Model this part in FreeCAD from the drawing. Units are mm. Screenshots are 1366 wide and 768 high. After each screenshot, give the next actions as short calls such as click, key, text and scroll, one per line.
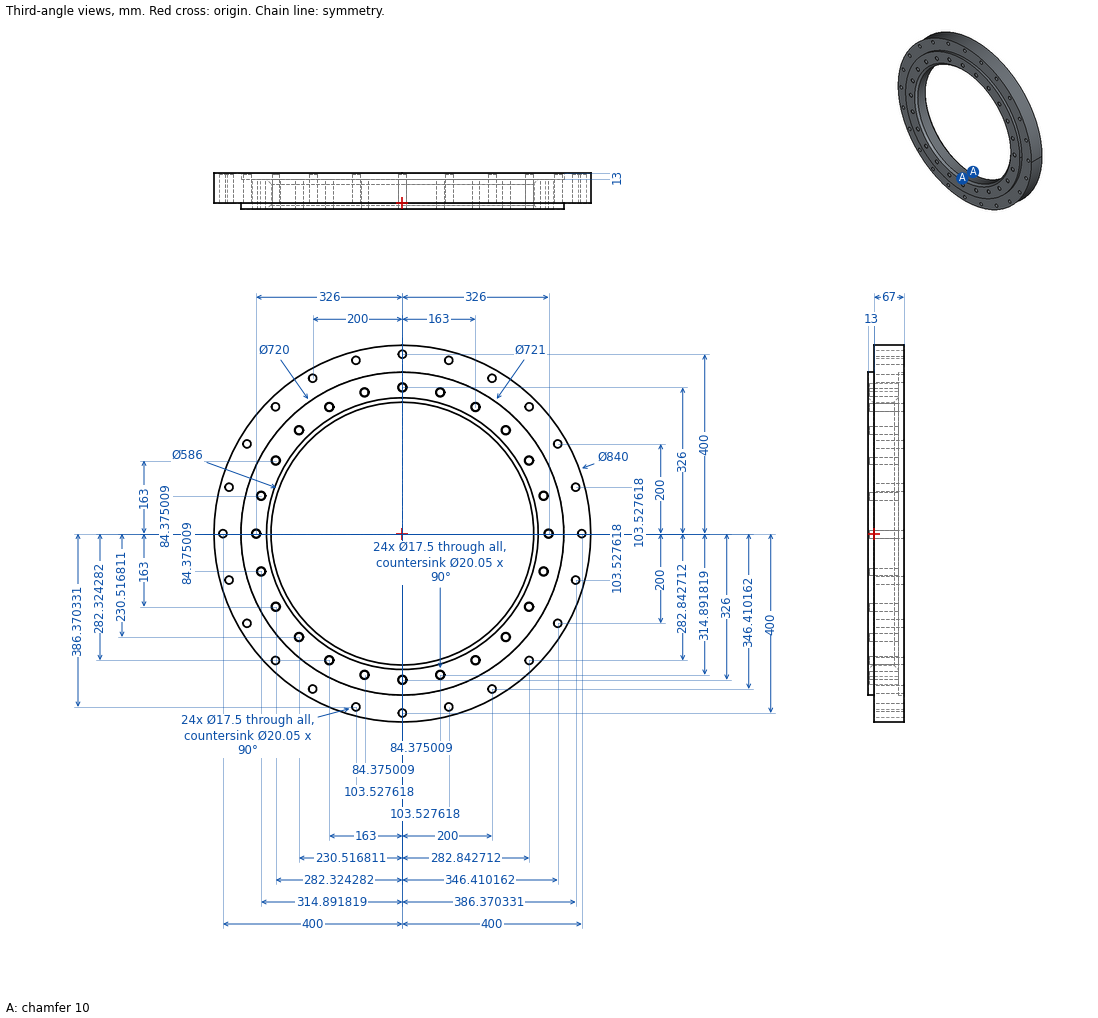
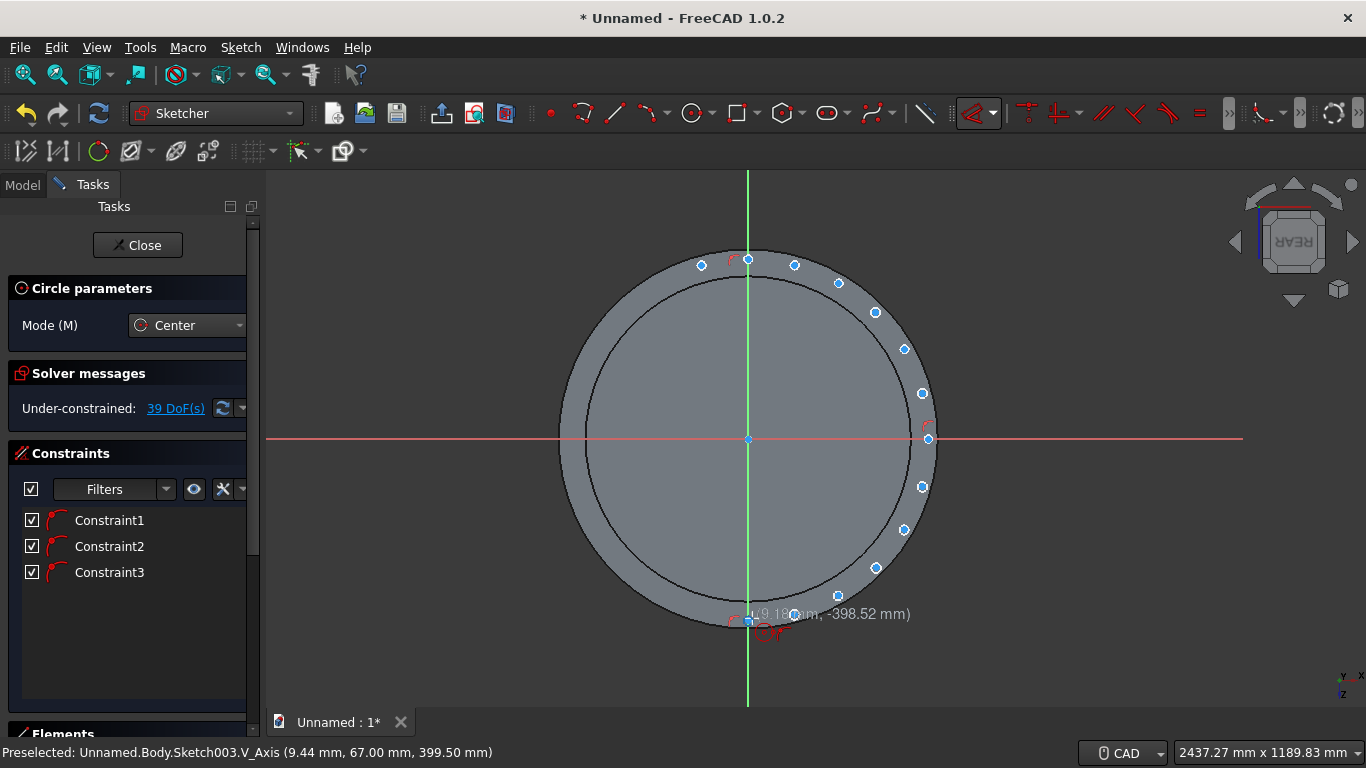
click(701, 613)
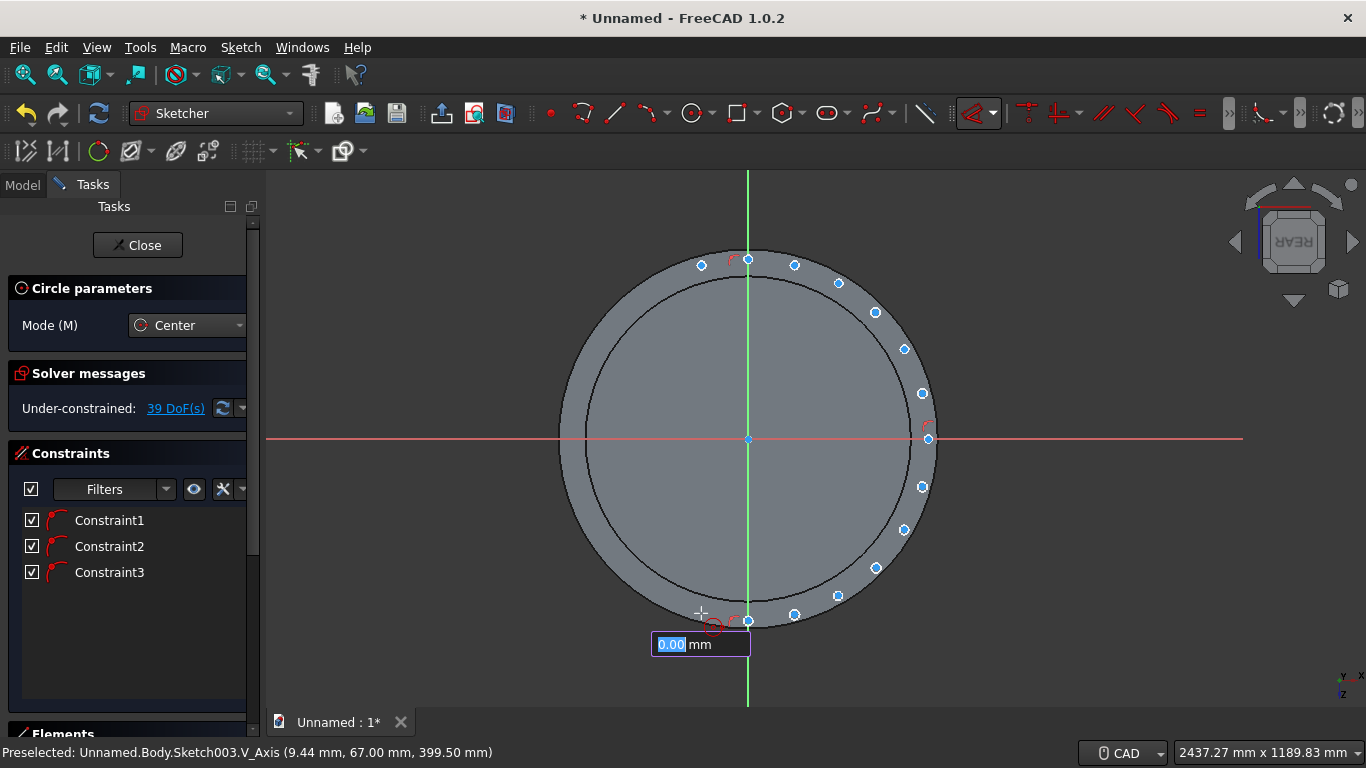
scroll(704, 611, up, 7)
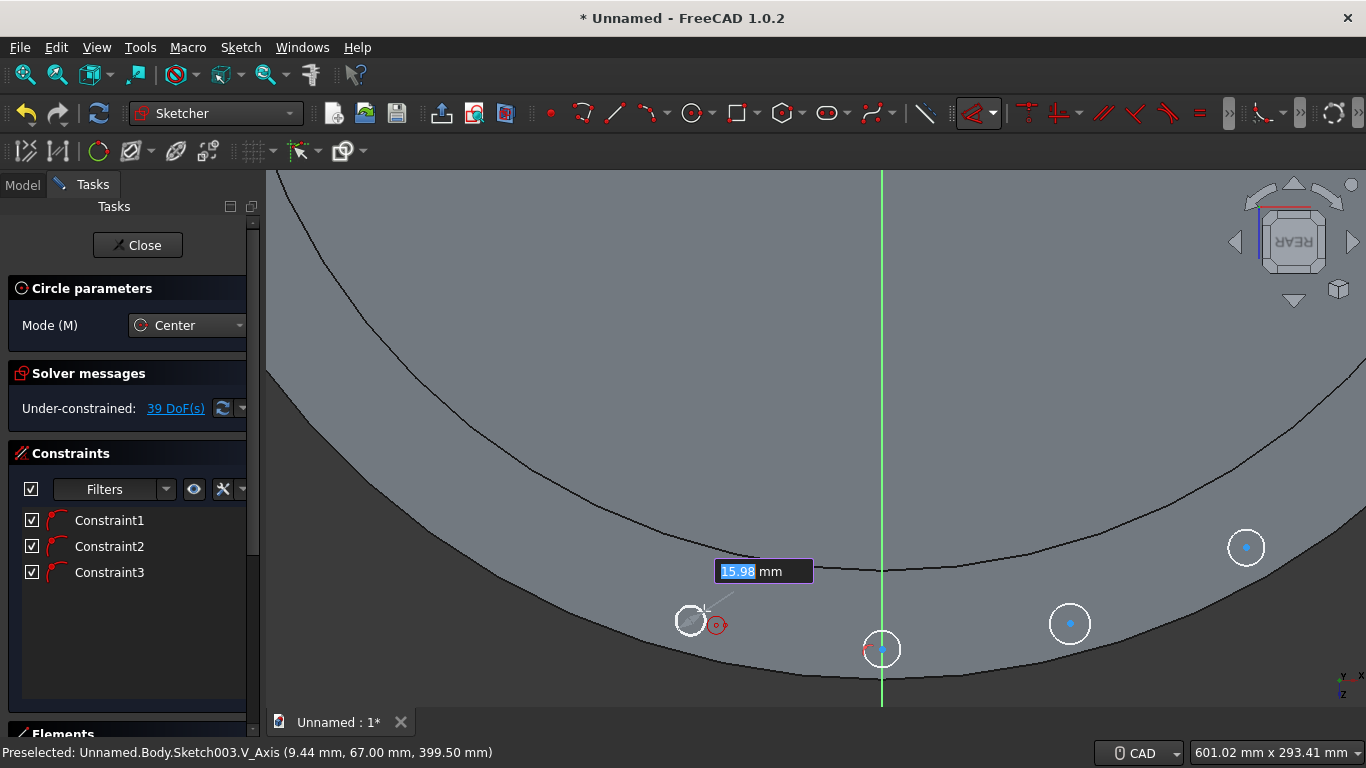
click(704, 607)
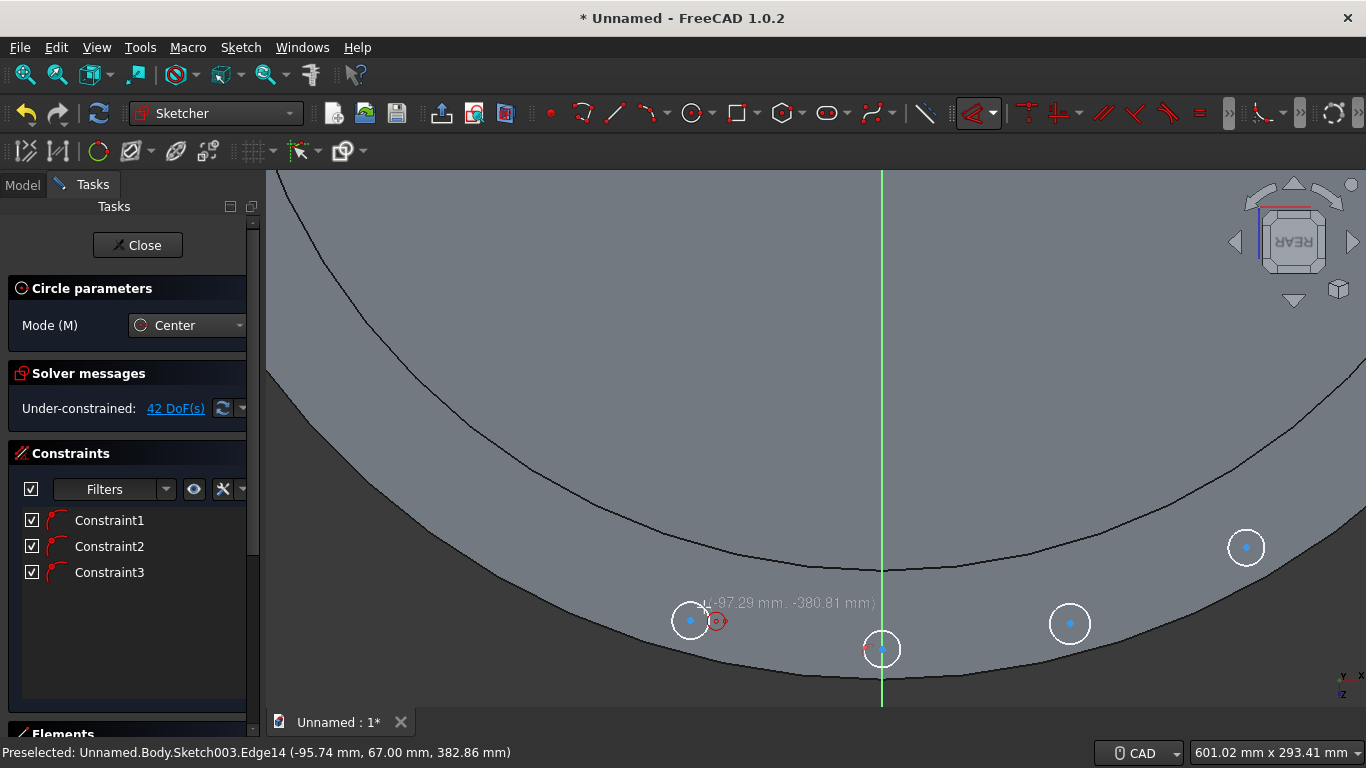
scroll(516, 545, up, 2)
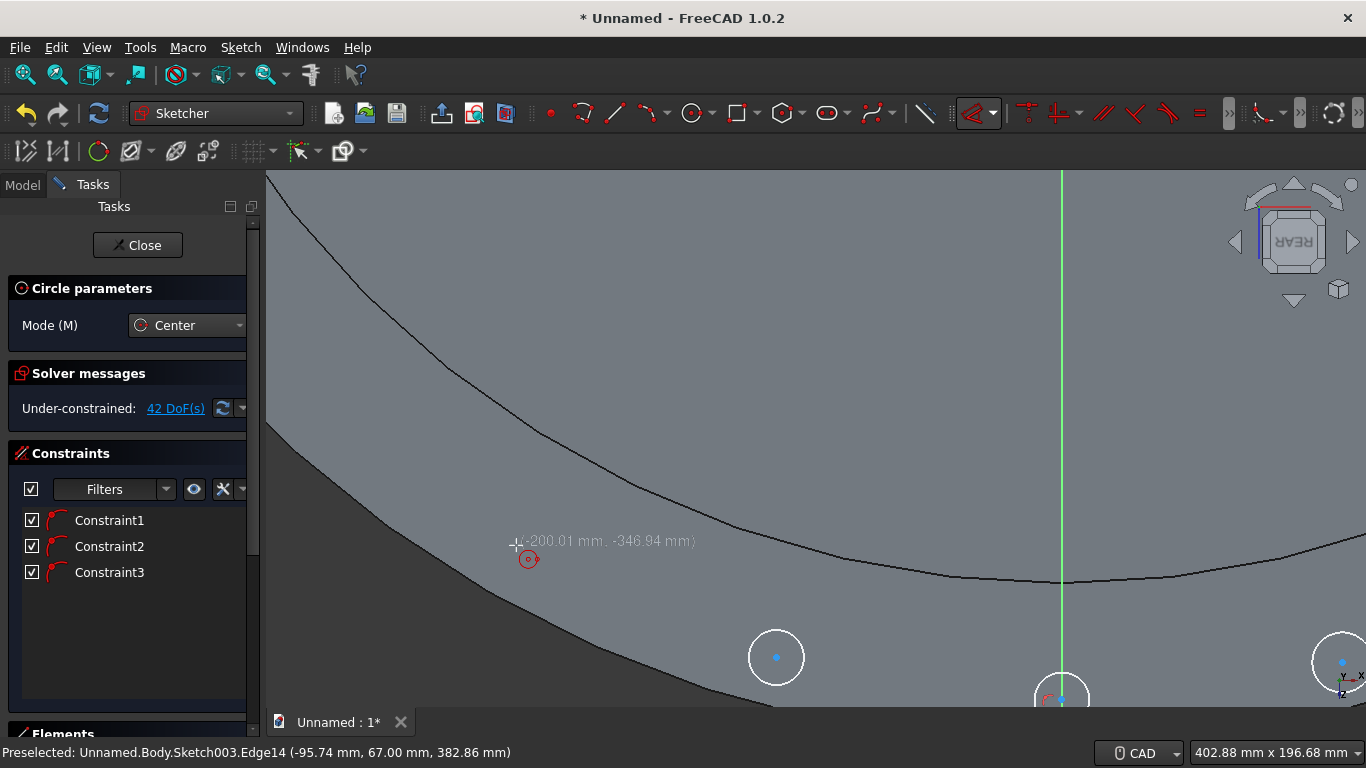
scroll(685, 605, down, 9)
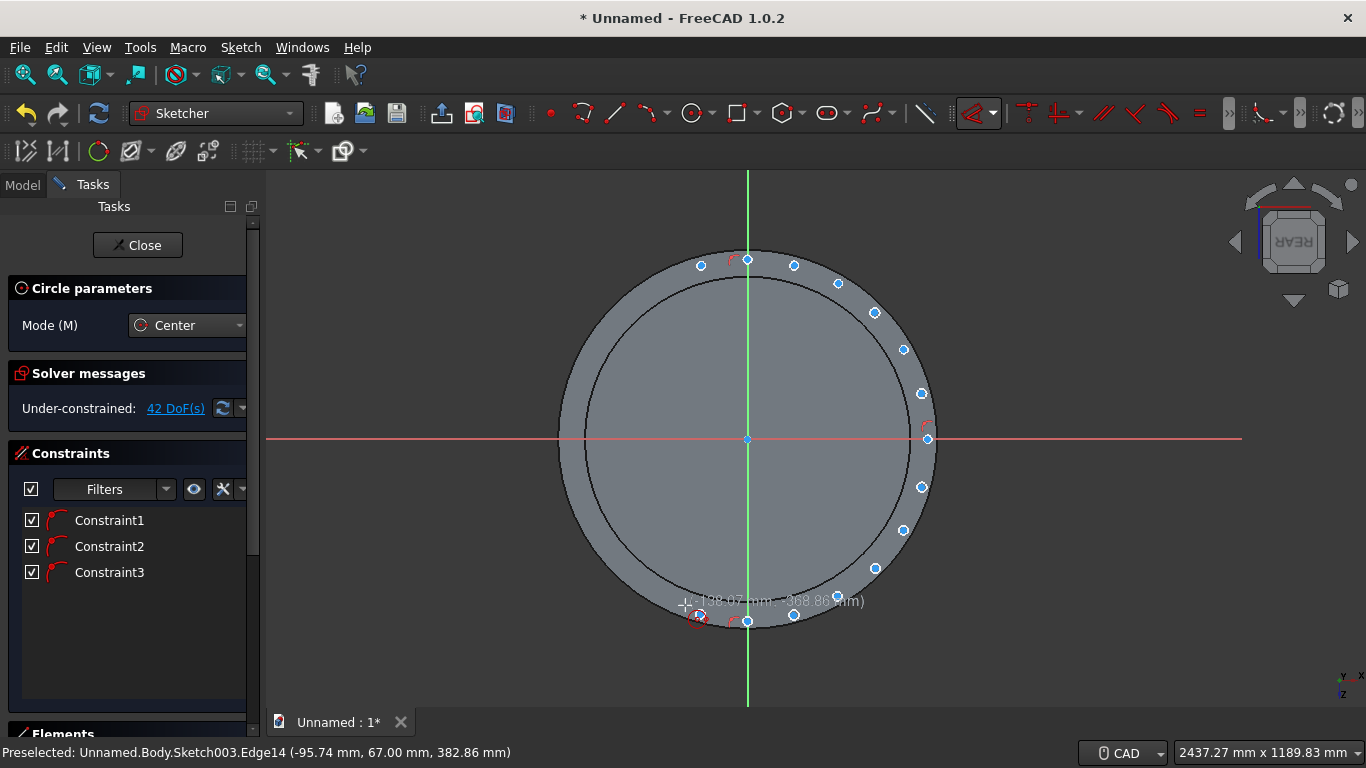
click(657, 596)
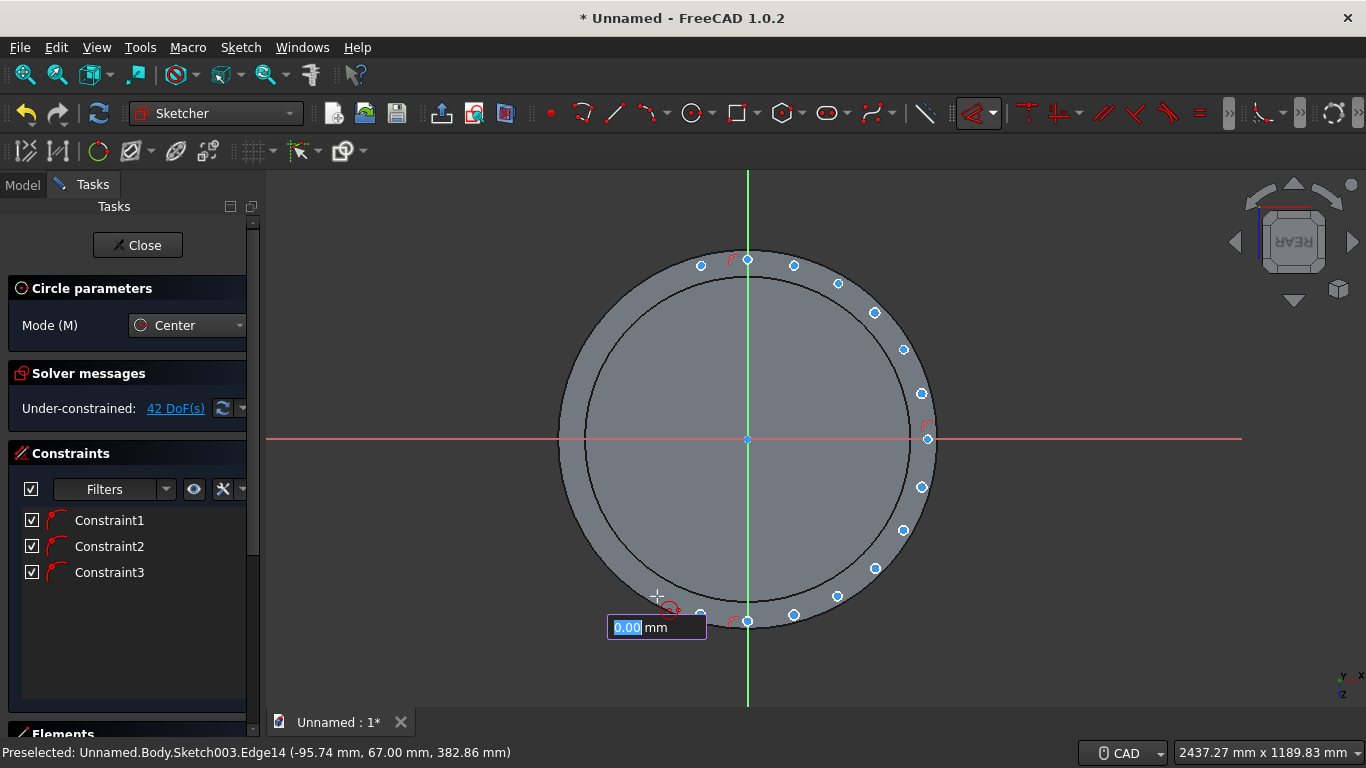
scroll(660, 593, up, 7)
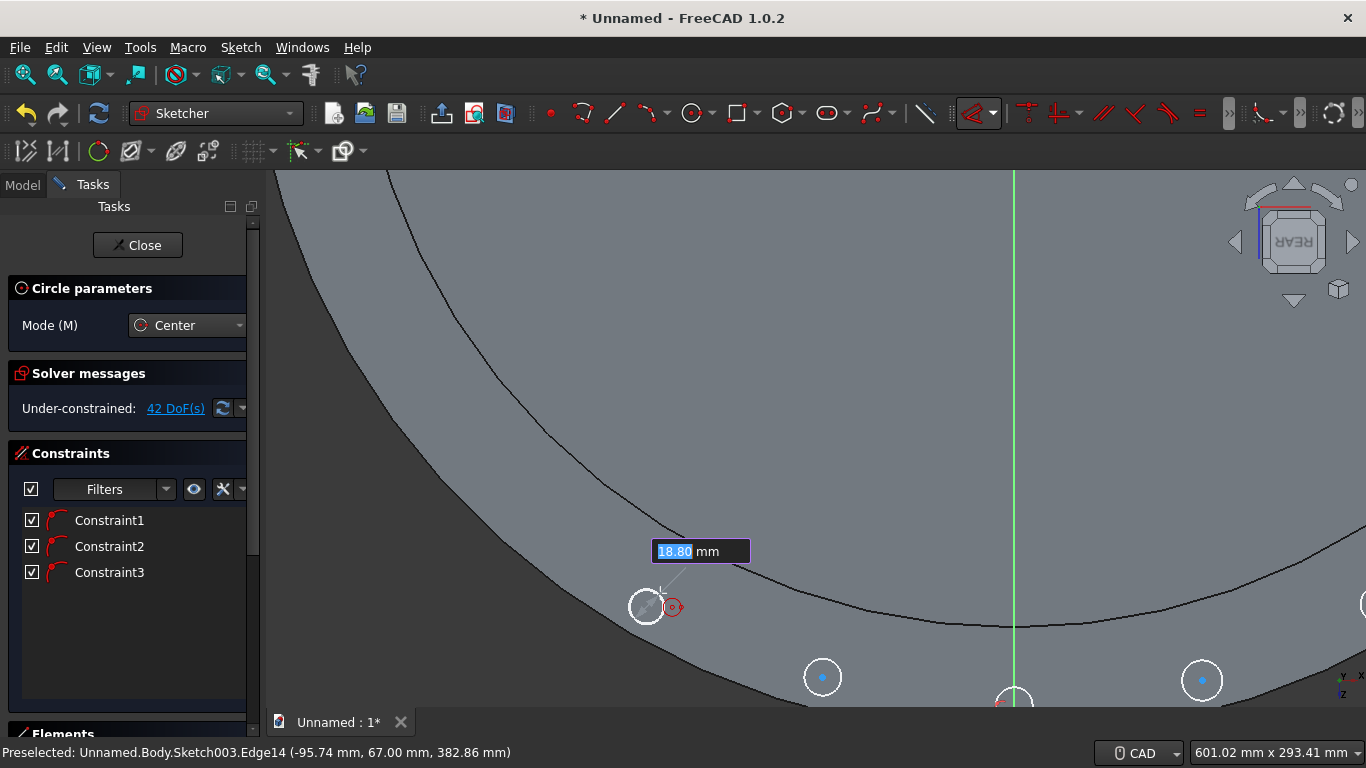
click(660, 590)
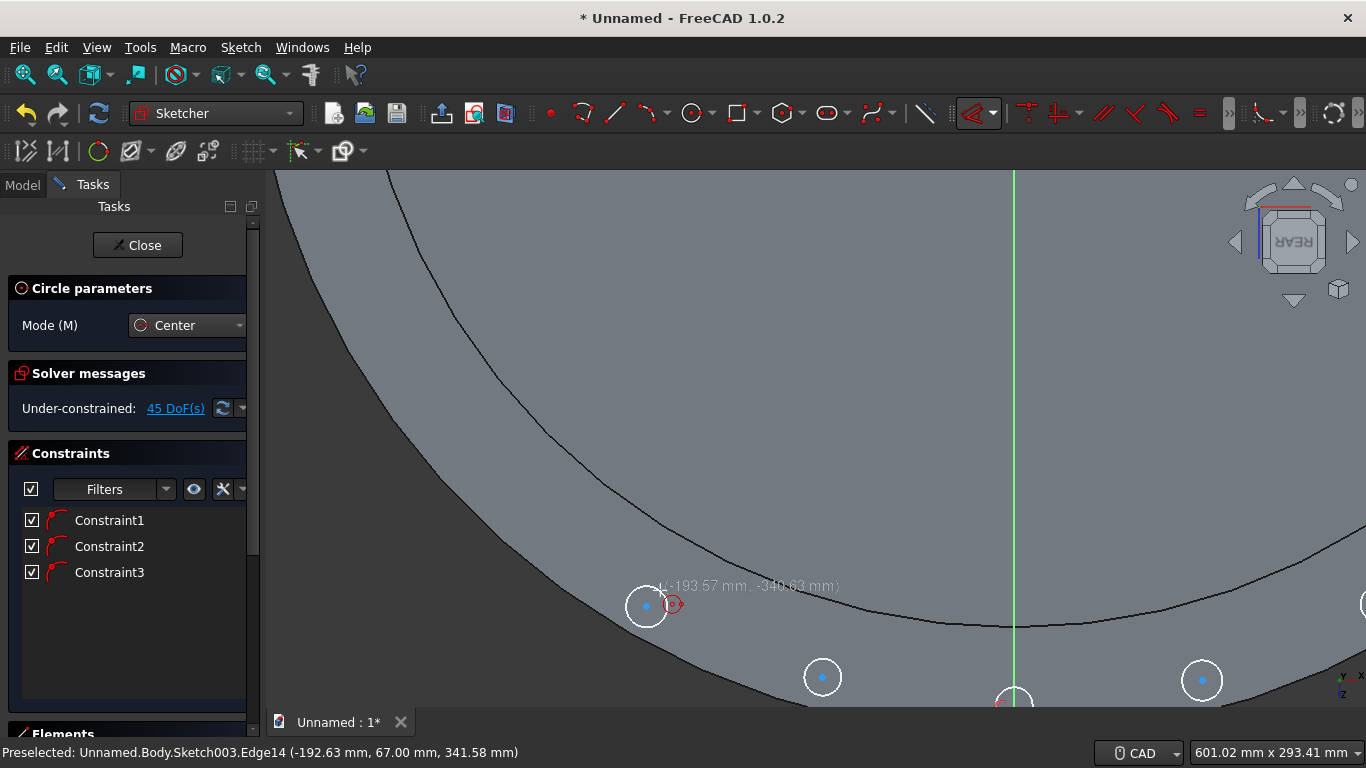
scroll(497, 485, up, 2)